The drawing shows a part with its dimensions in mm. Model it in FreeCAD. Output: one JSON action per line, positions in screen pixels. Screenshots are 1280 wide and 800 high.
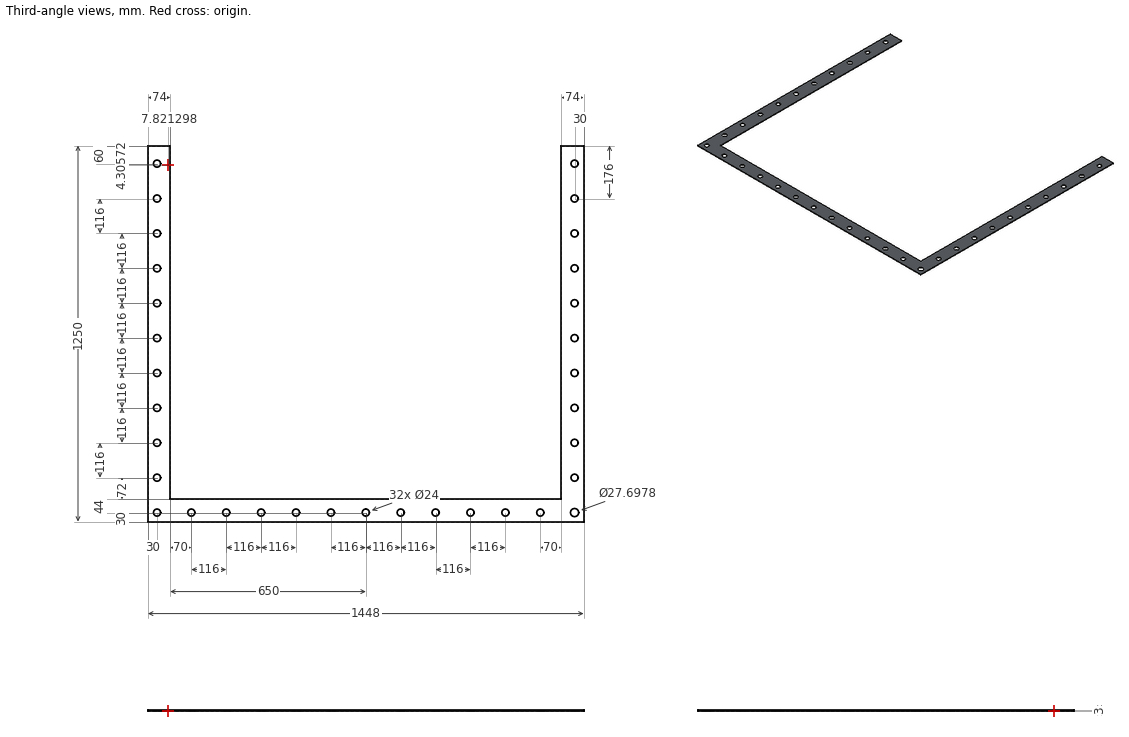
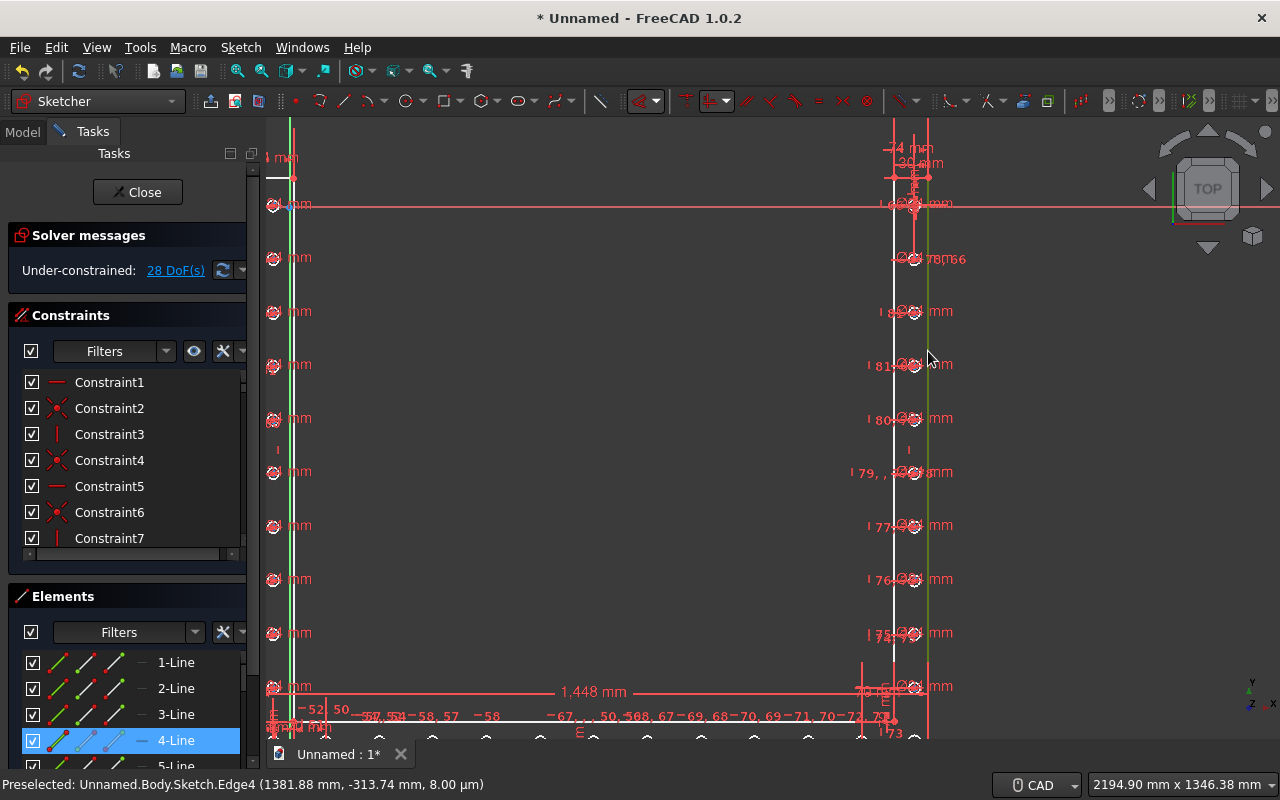
{"action": "left_click", "coordinate": [658, 102]}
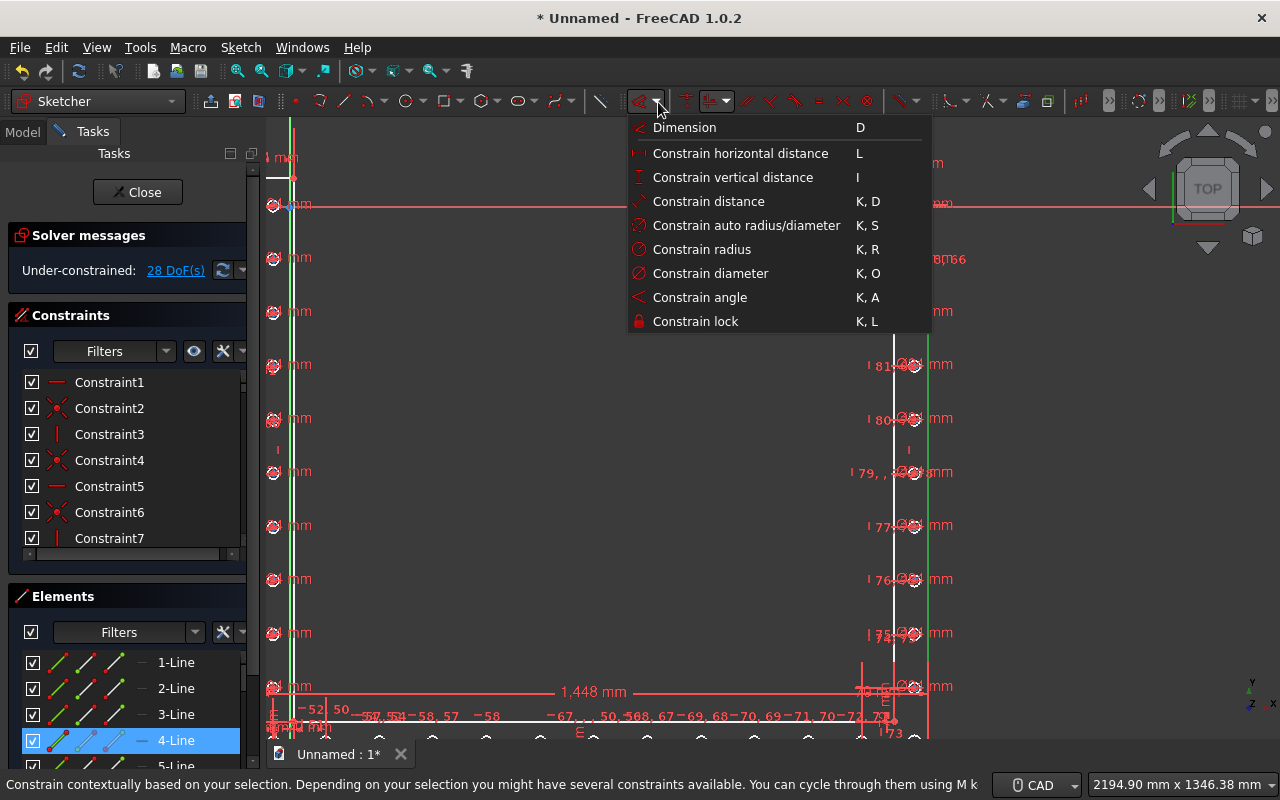
{"action": "left_click", "coordinate": [780, 177]}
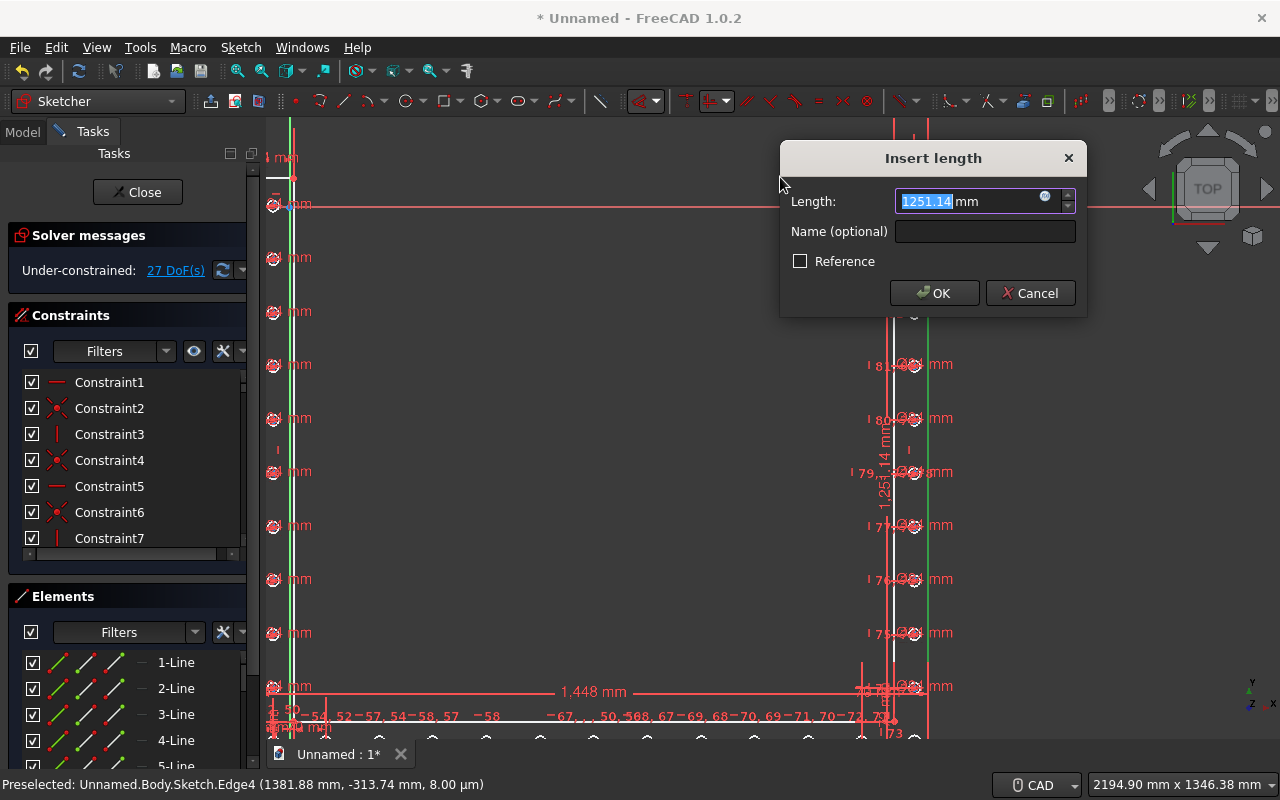
{"action": "type", "text": "1250"}
{"action": "key", "text": "Return"}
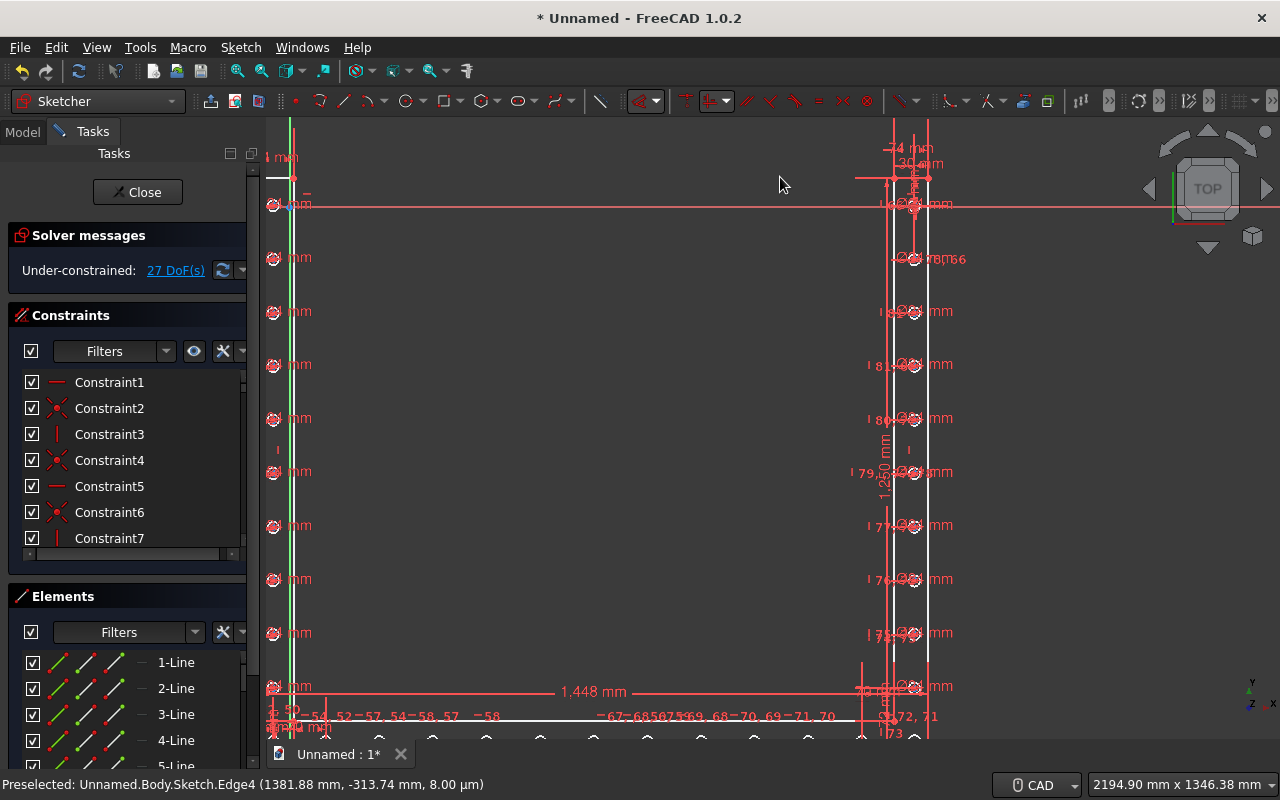
{"action": "scroll", "coordinate": [930, 351], "scroll_direction": "down", "scroll_amount": 2}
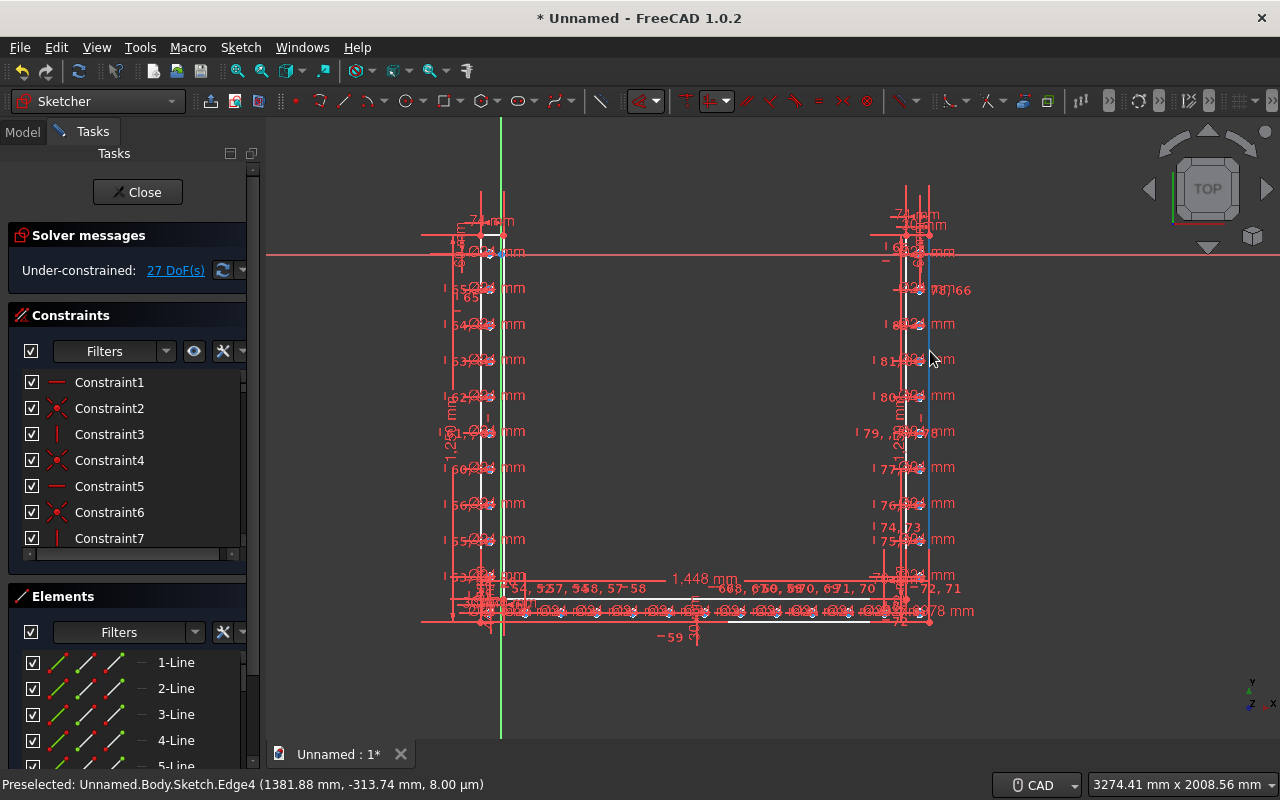
{"action": "left_click", "coordinate": [504, 599]}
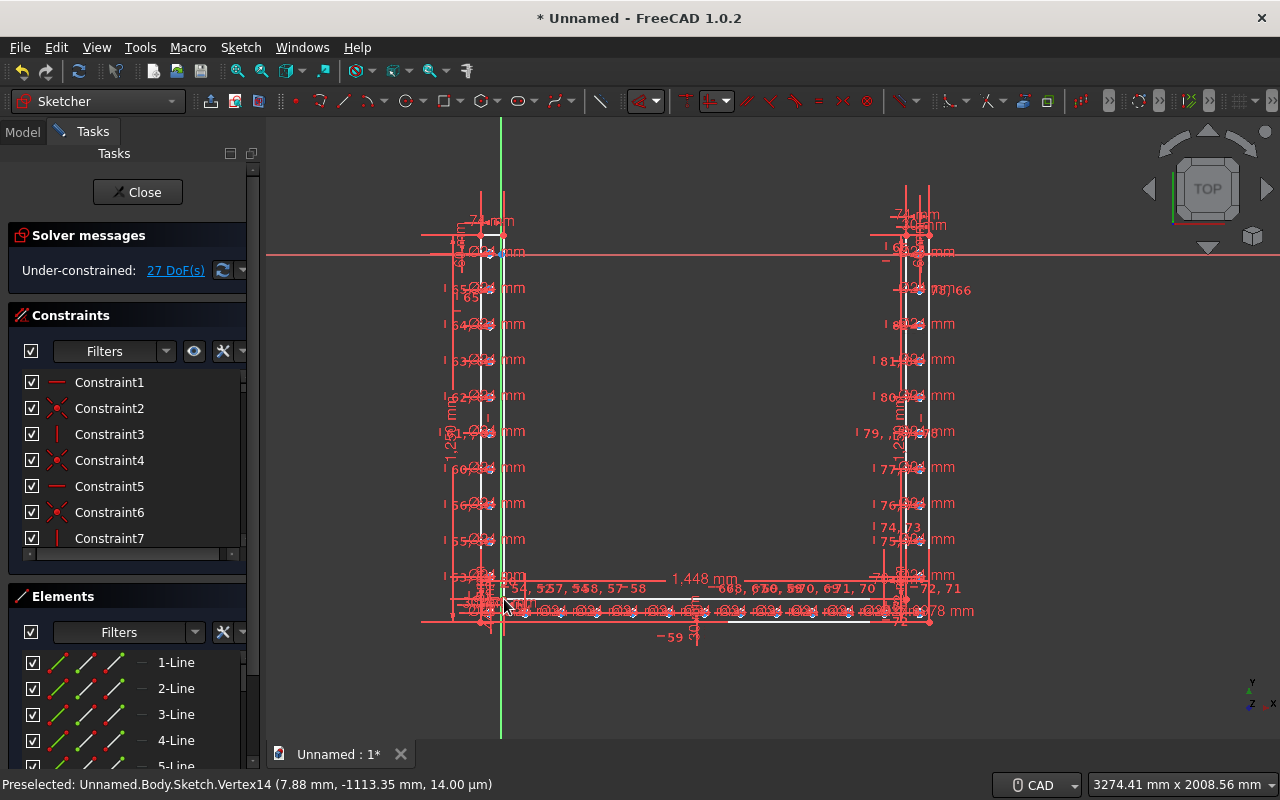
{"action": "left_click", "coordinate": [705, 613]}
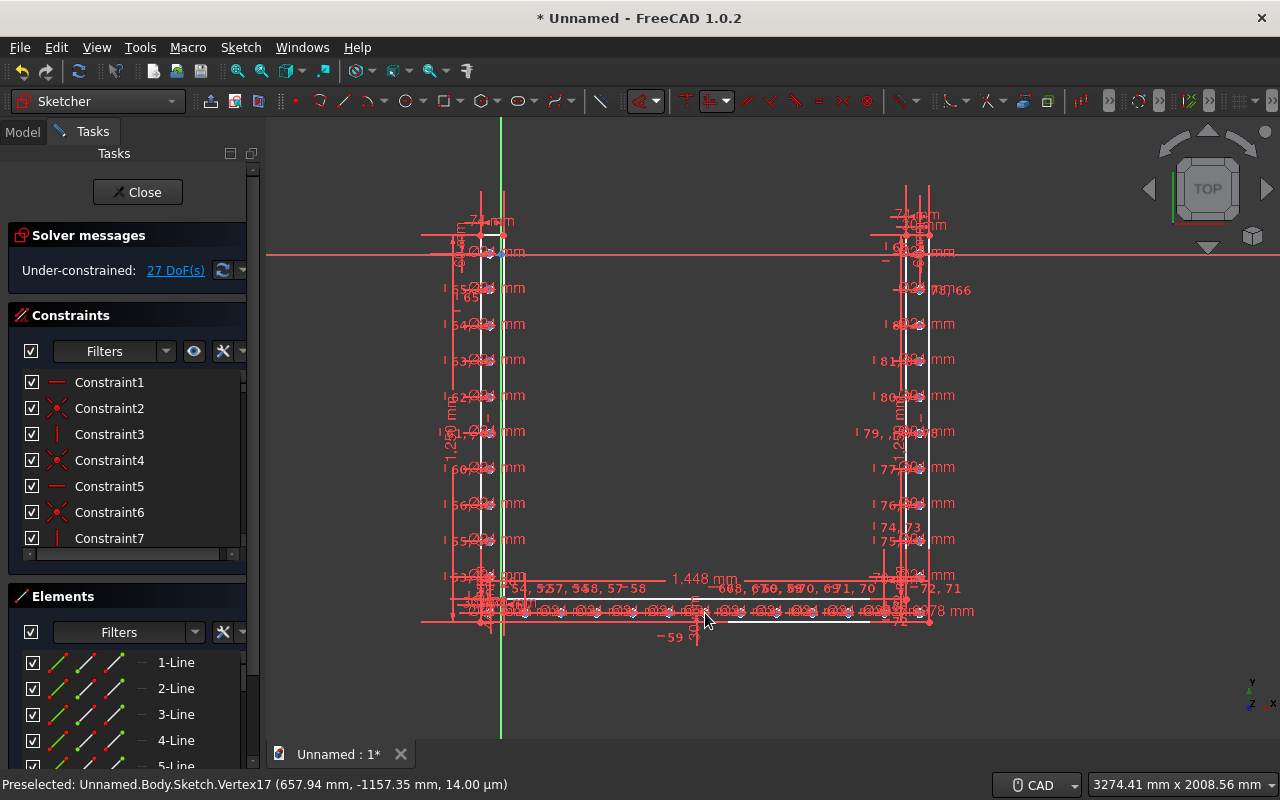
{"action": "key", "text": "l"}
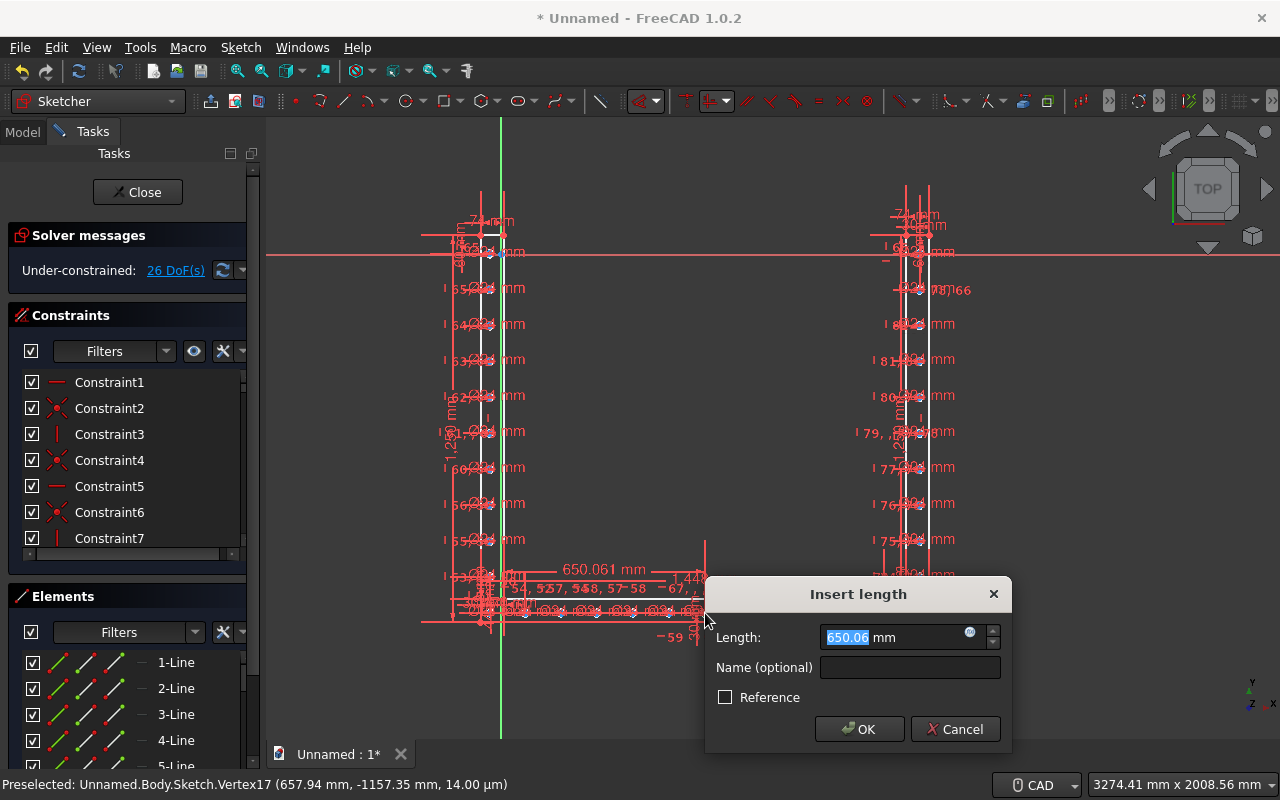
{"action": "type", "text": "650"}
{"action": "key", "text": "Return"}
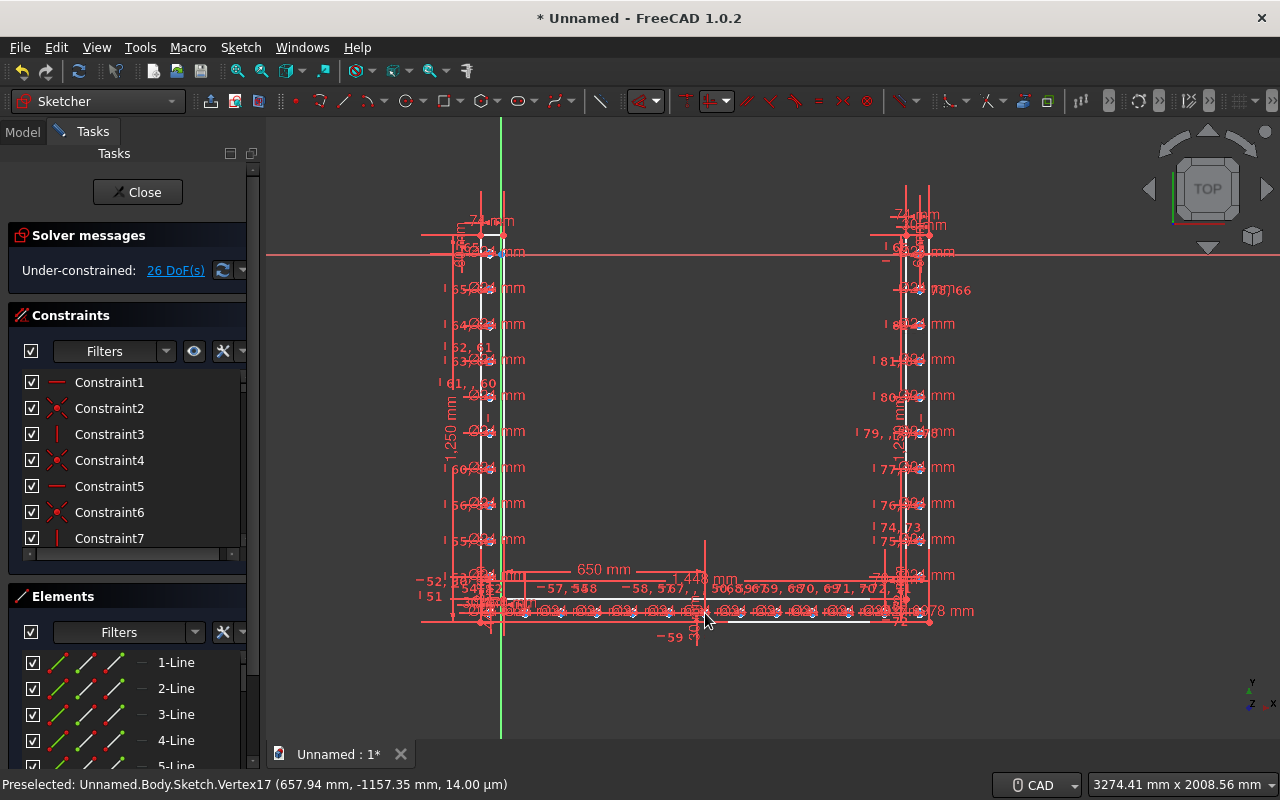
{"action": "left_click", "coordinate": [490, 577]}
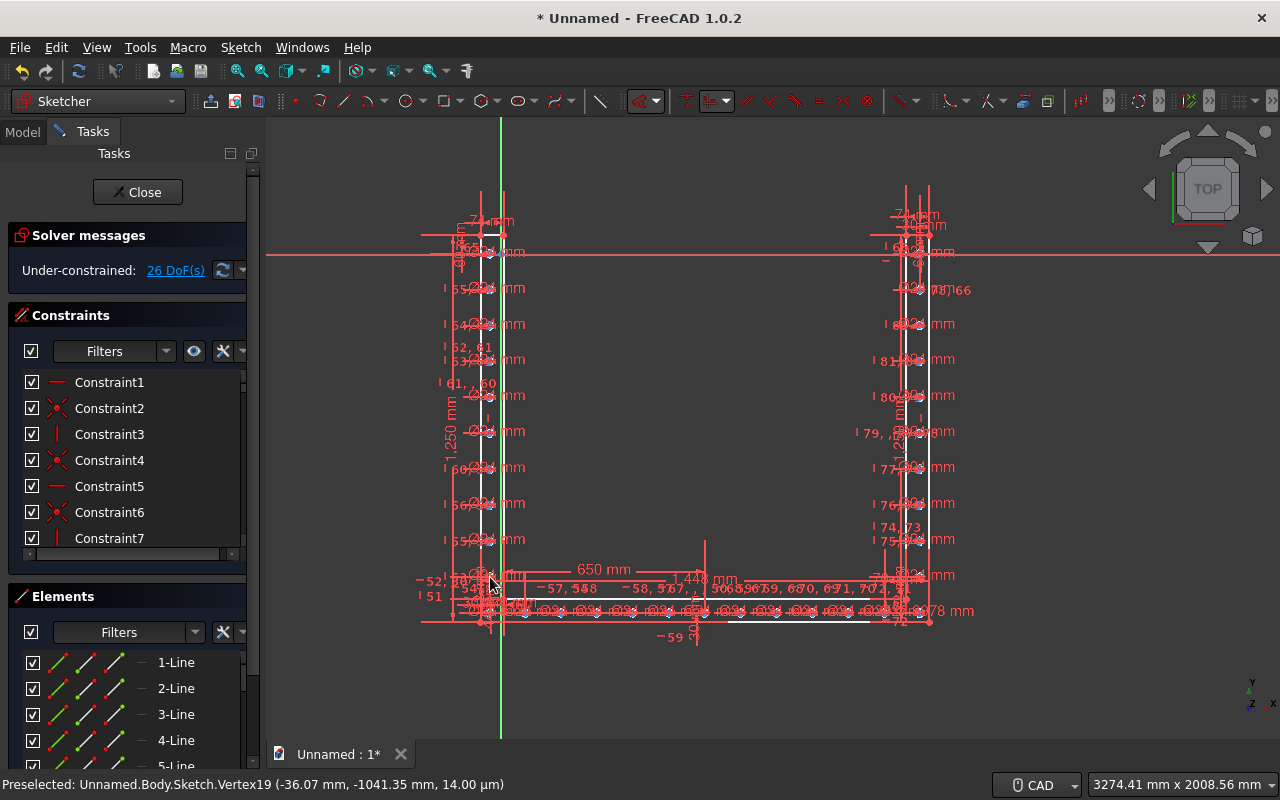
{"action": "left_click", "coordinate": [490, 541]}